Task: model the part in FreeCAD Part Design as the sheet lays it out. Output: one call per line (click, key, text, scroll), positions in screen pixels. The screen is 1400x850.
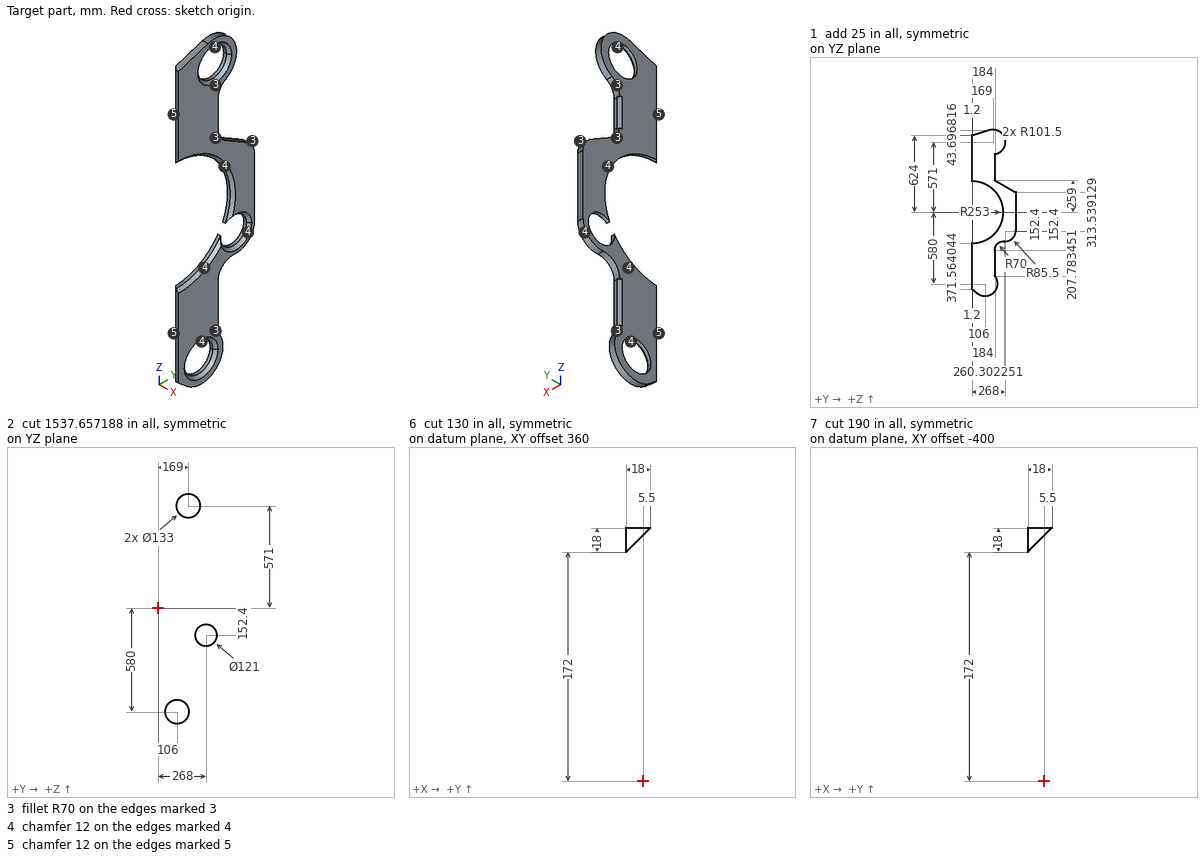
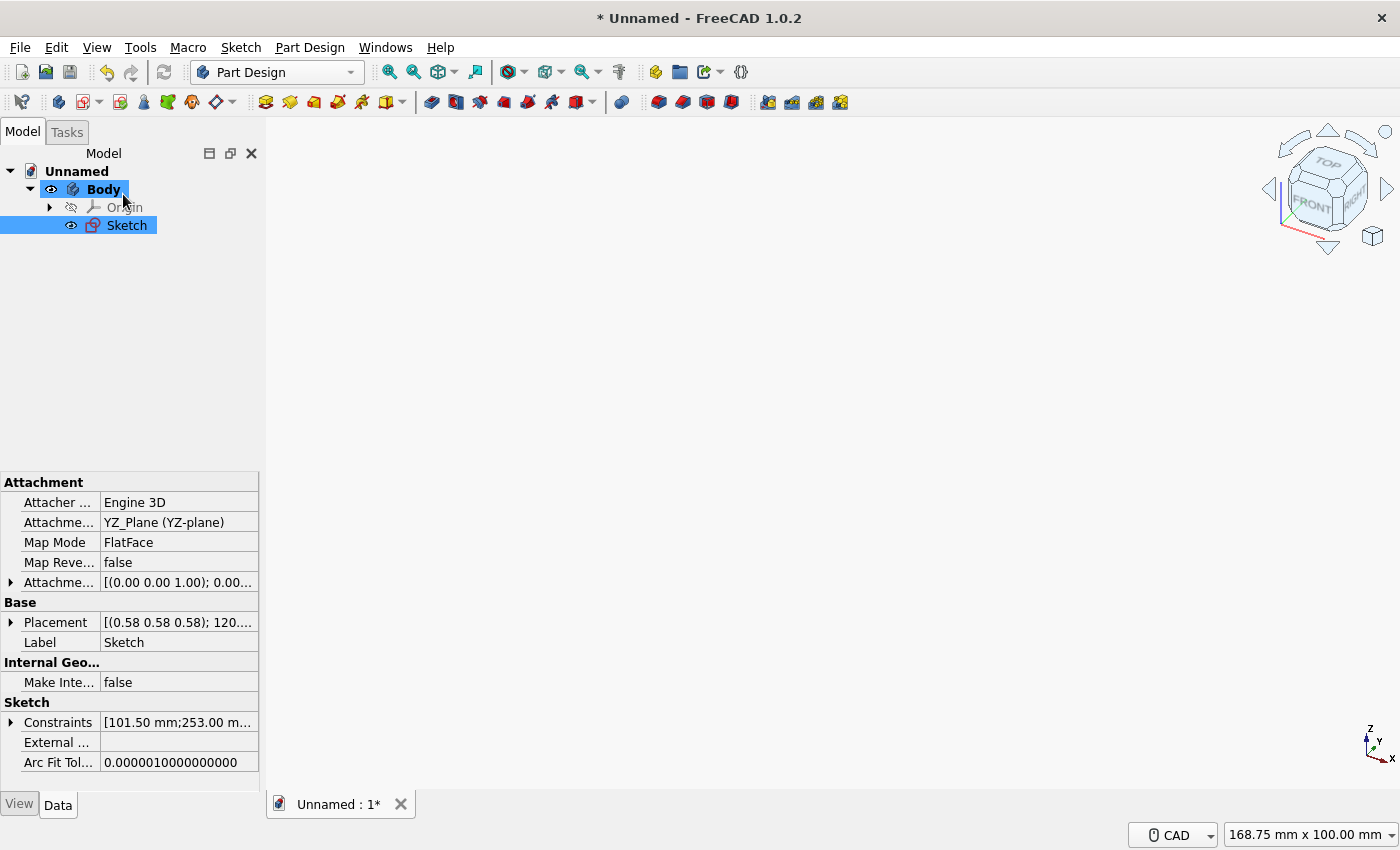
click(266, 102)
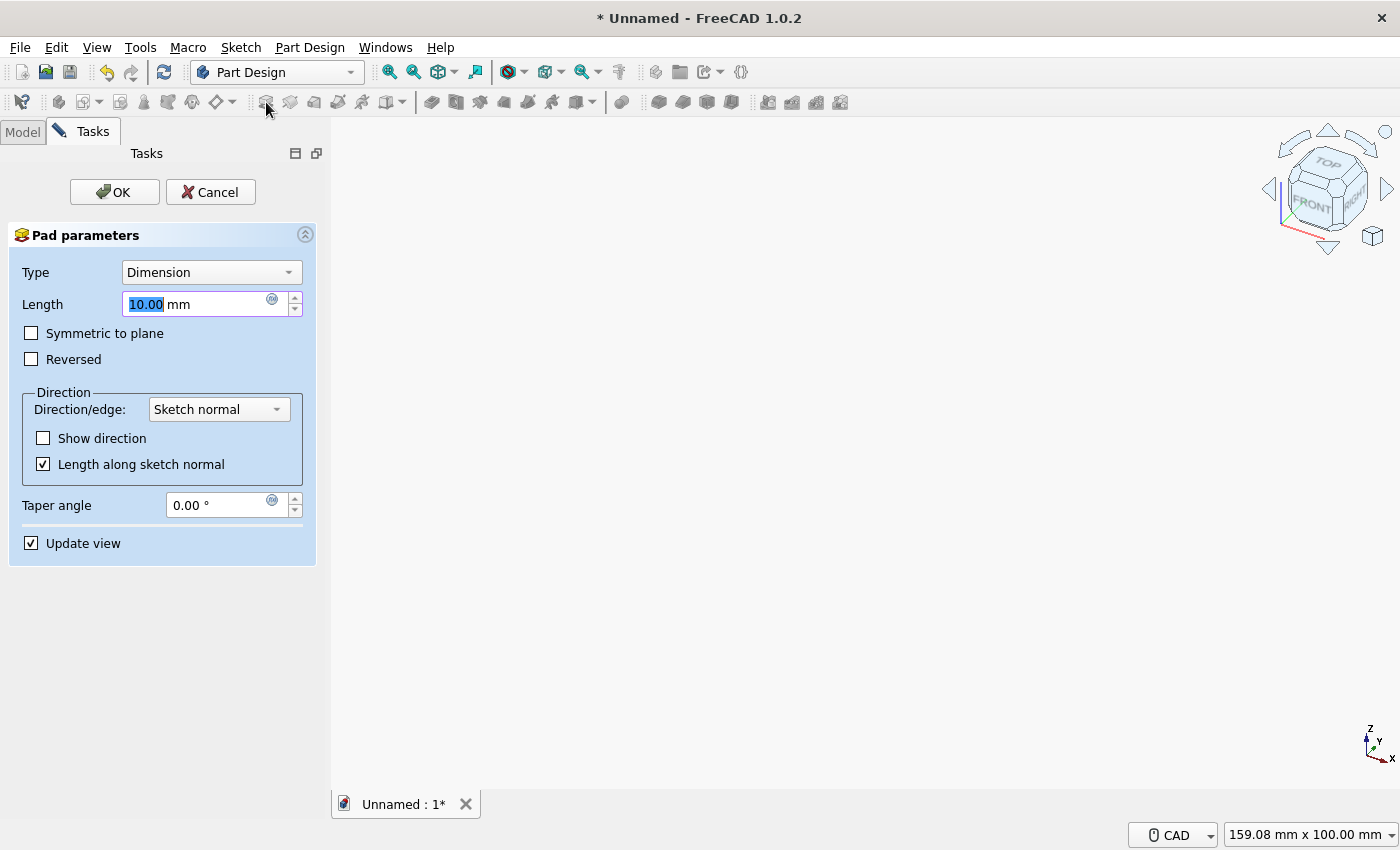
text(25)
key(Tab)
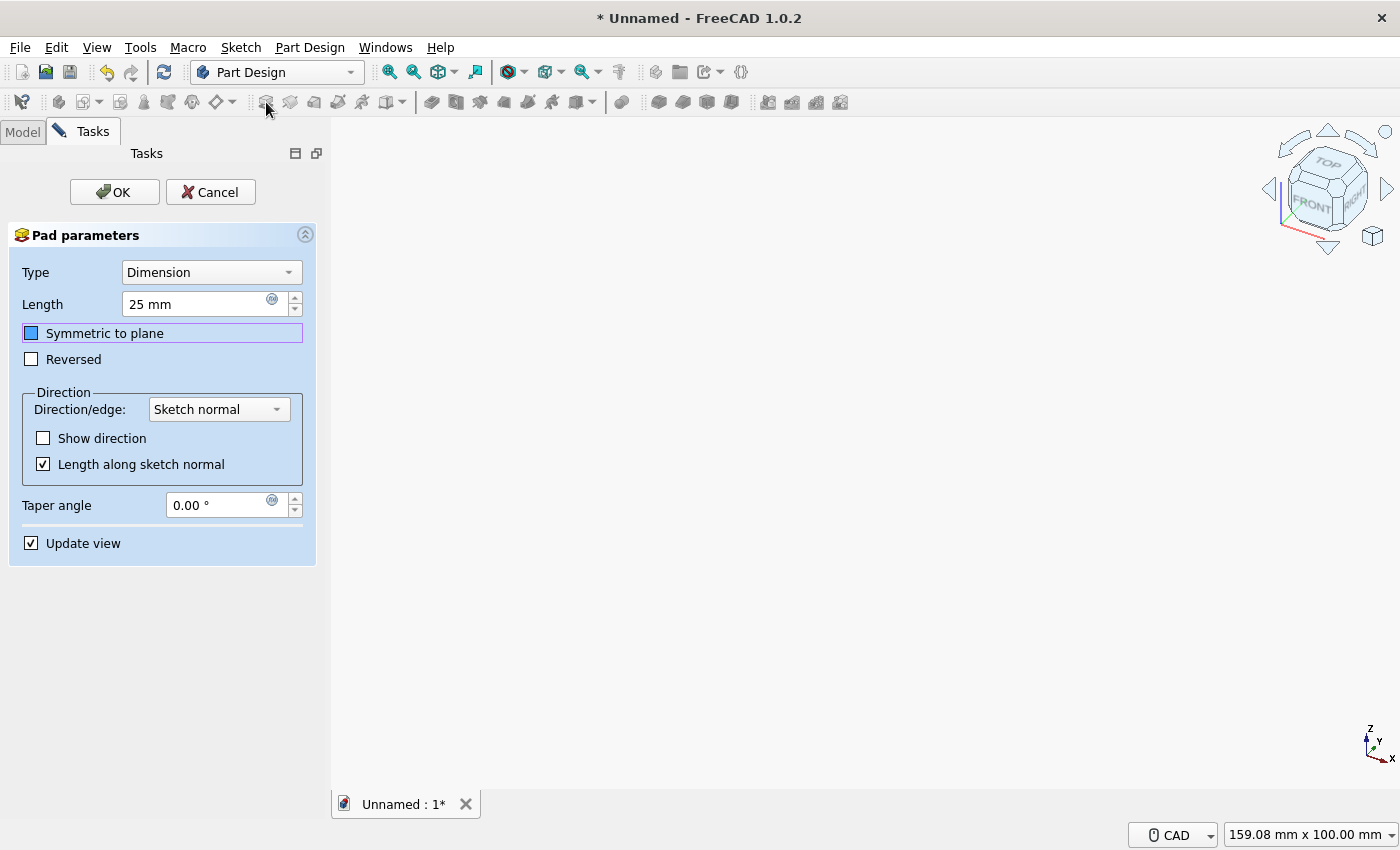
click(30, 333)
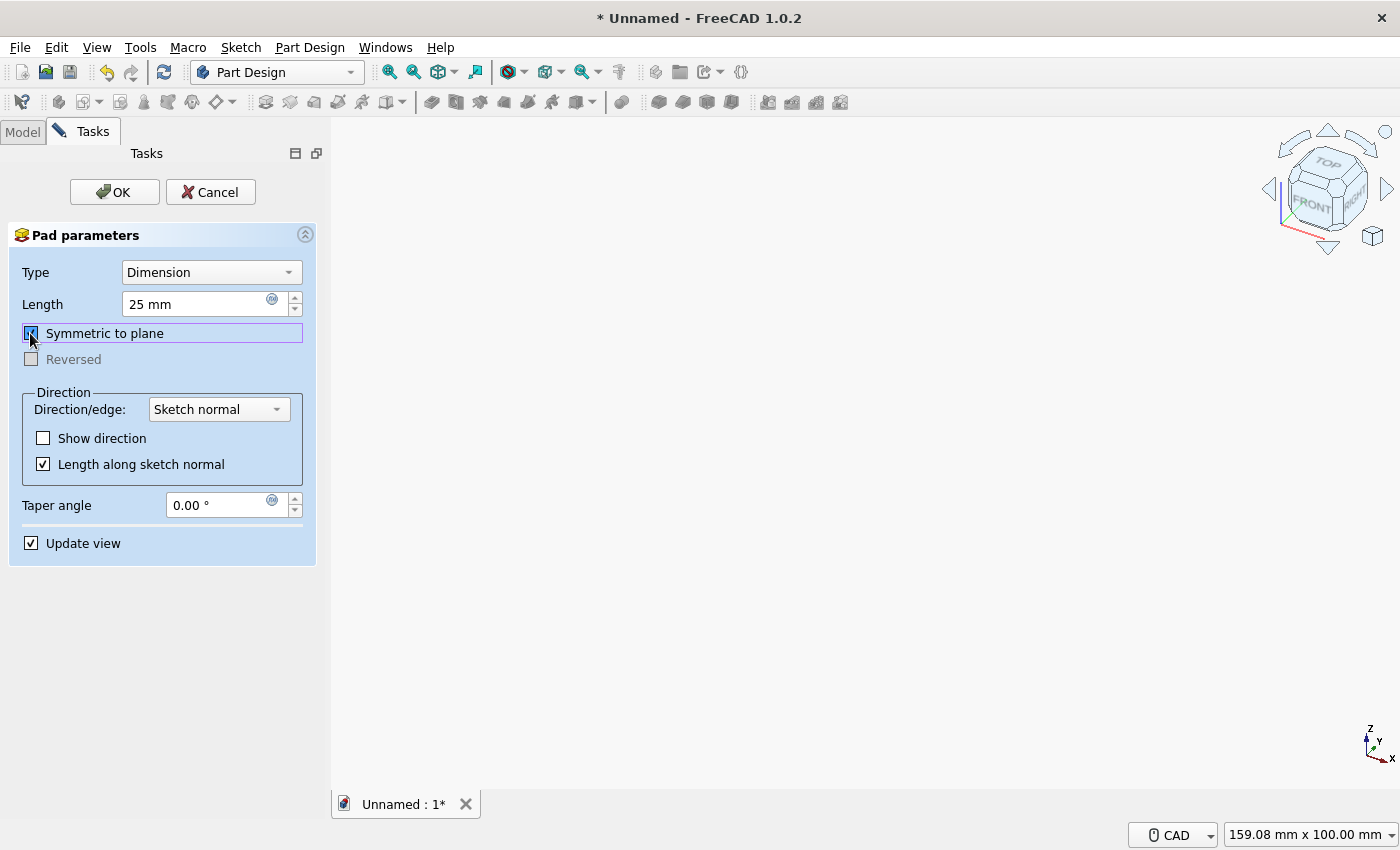
click(115, 192)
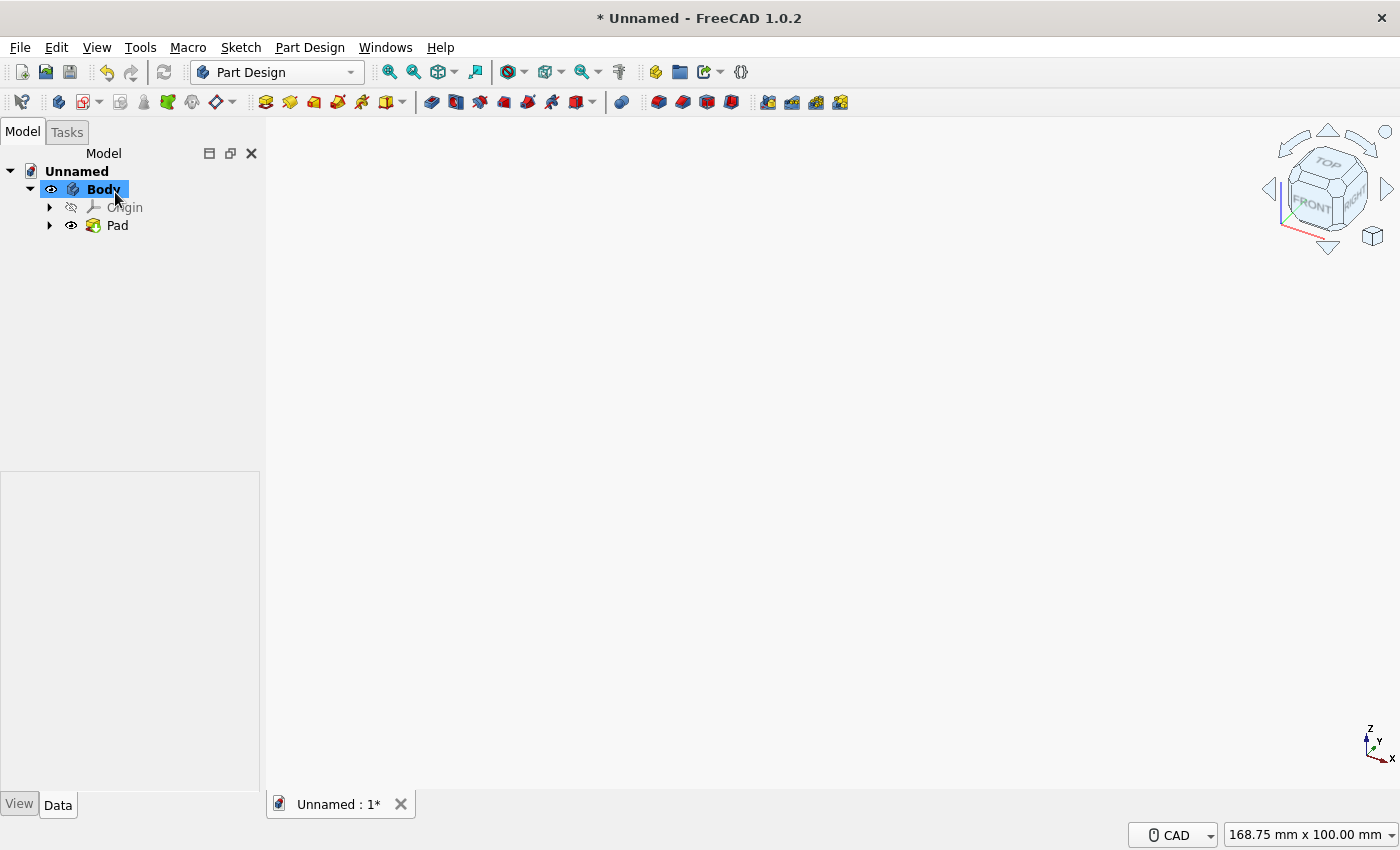
click(390, 72)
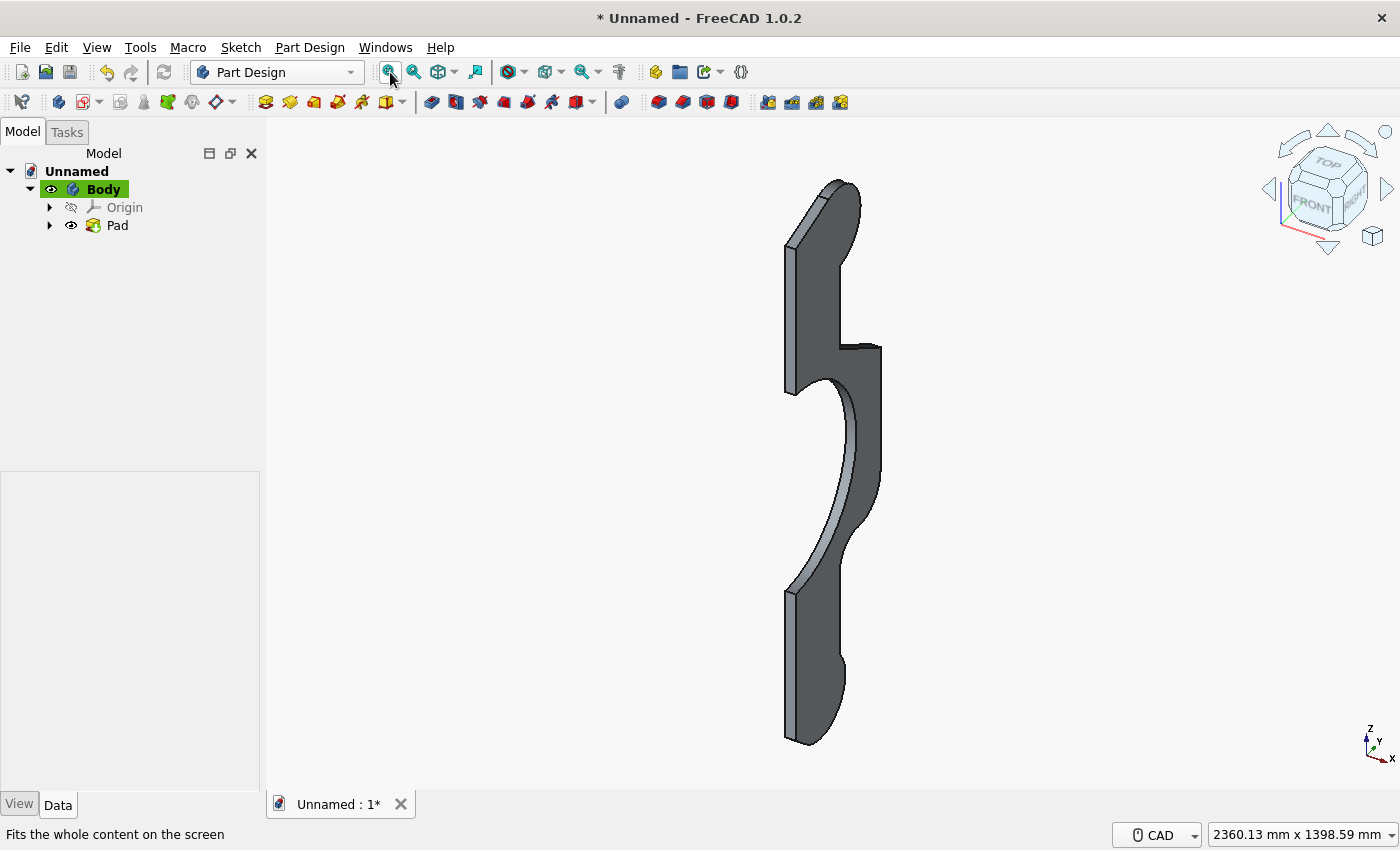
click(84, 102)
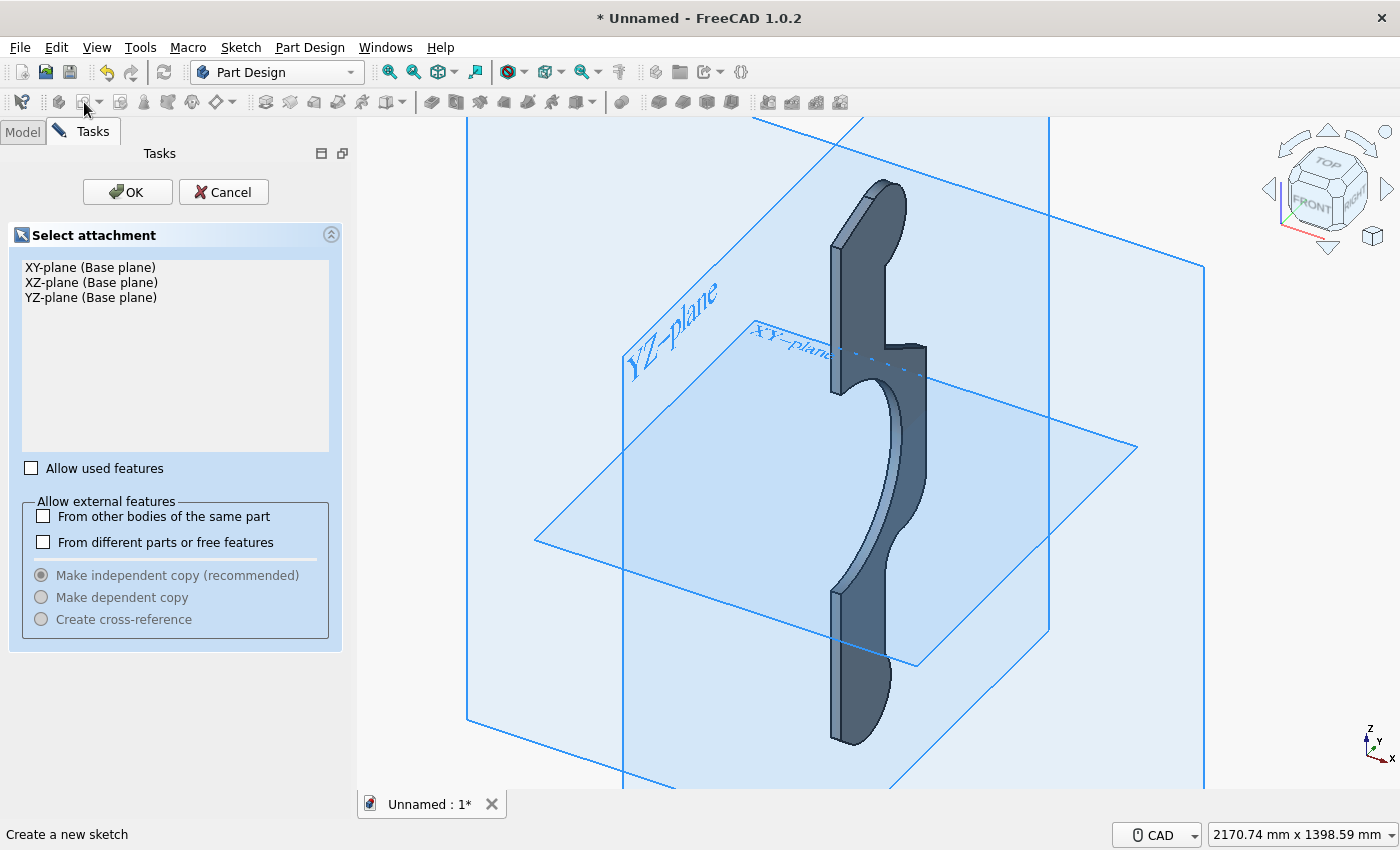
click(82, 298)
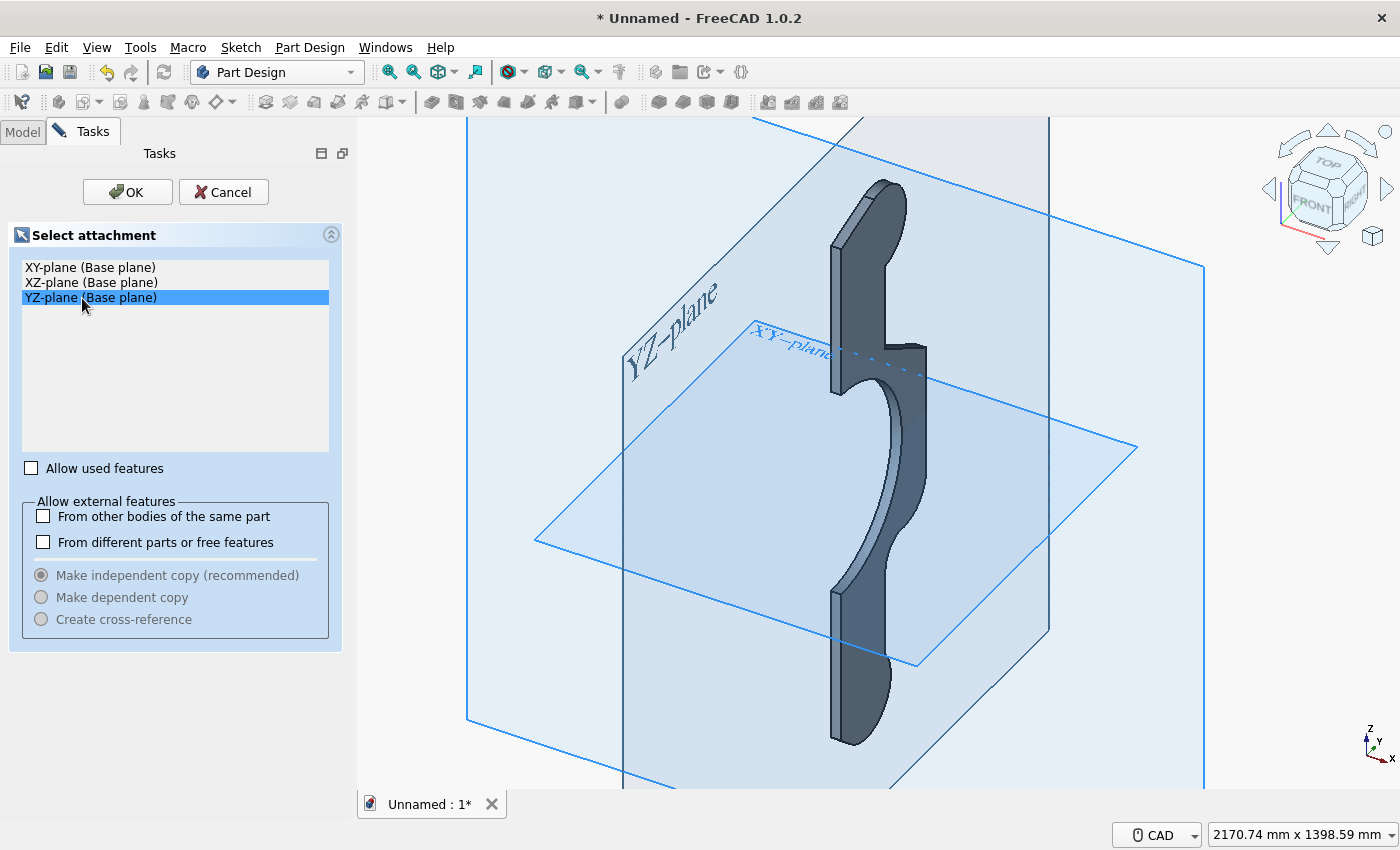
click(128, 192)